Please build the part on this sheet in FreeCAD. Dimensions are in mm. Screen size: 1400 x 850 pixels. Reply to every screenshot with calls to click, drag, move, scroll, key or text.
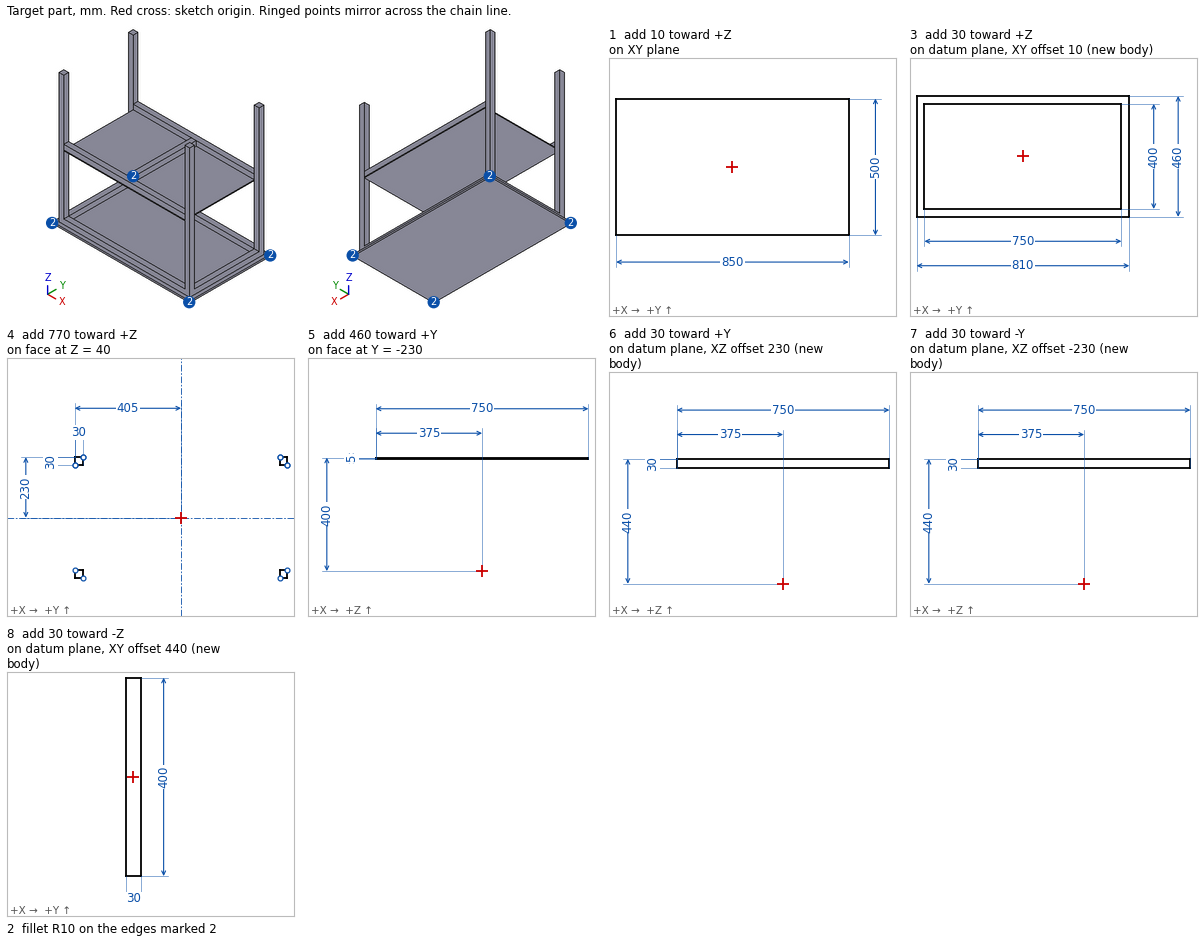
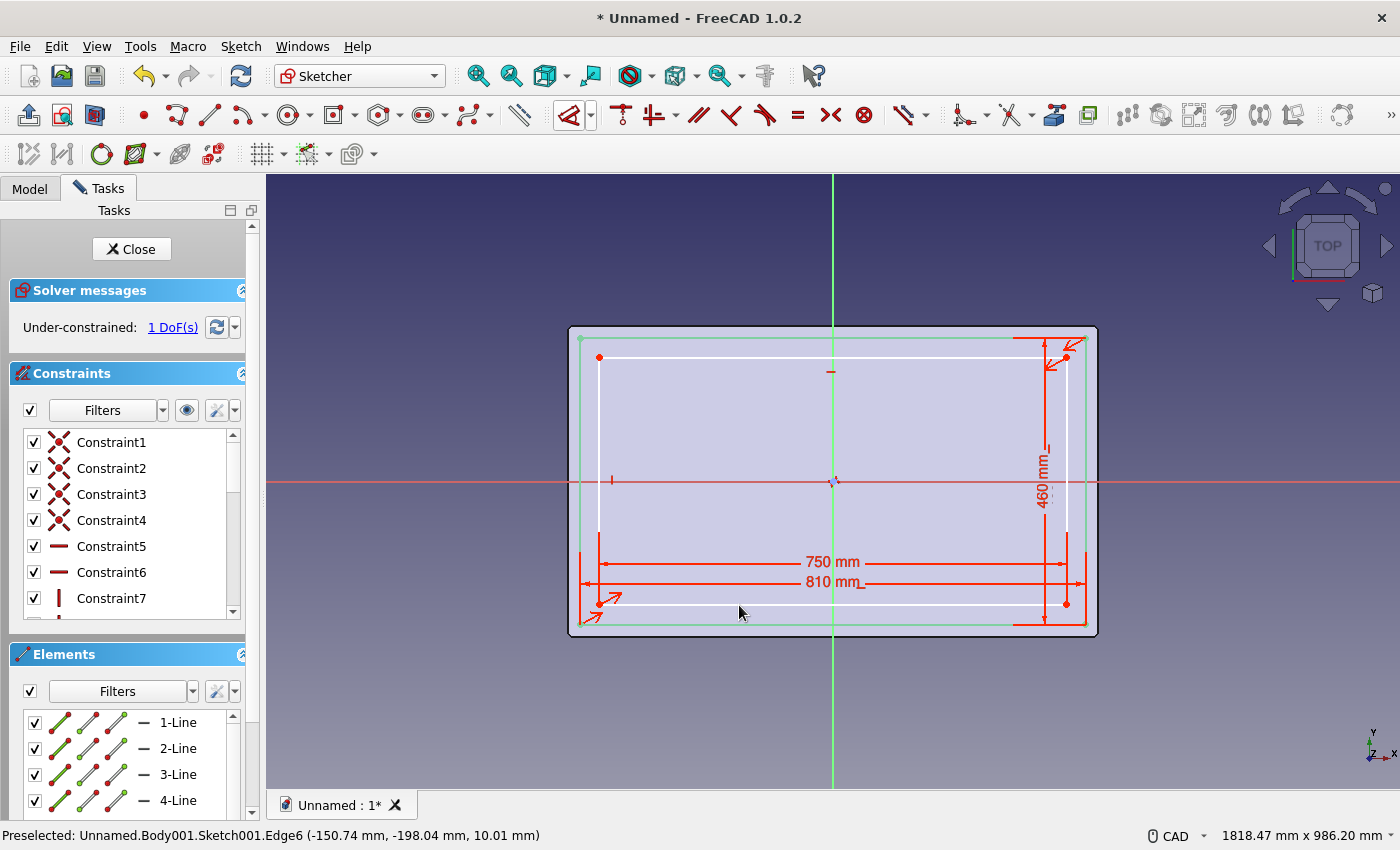
click(1067, 531)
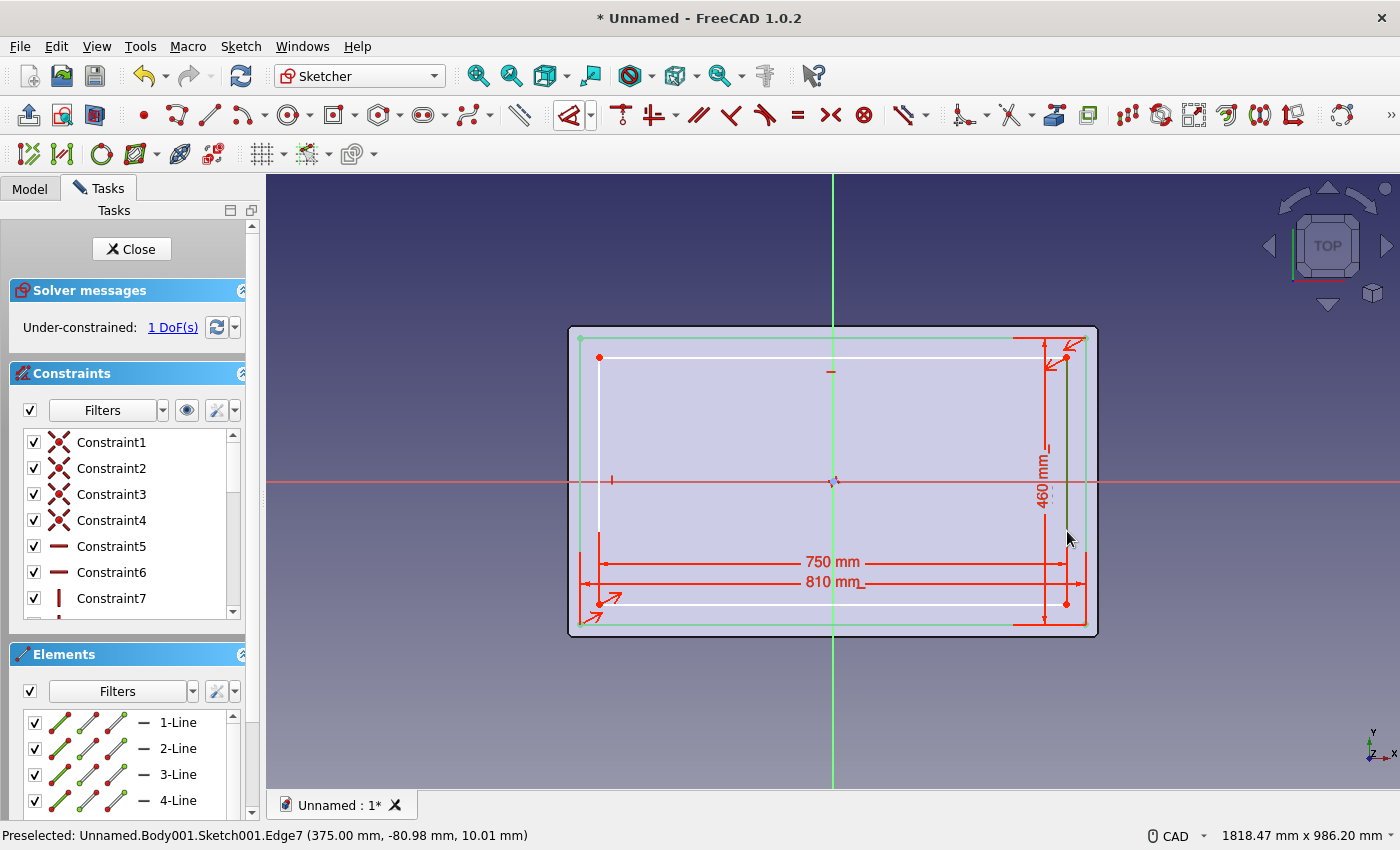
key(i)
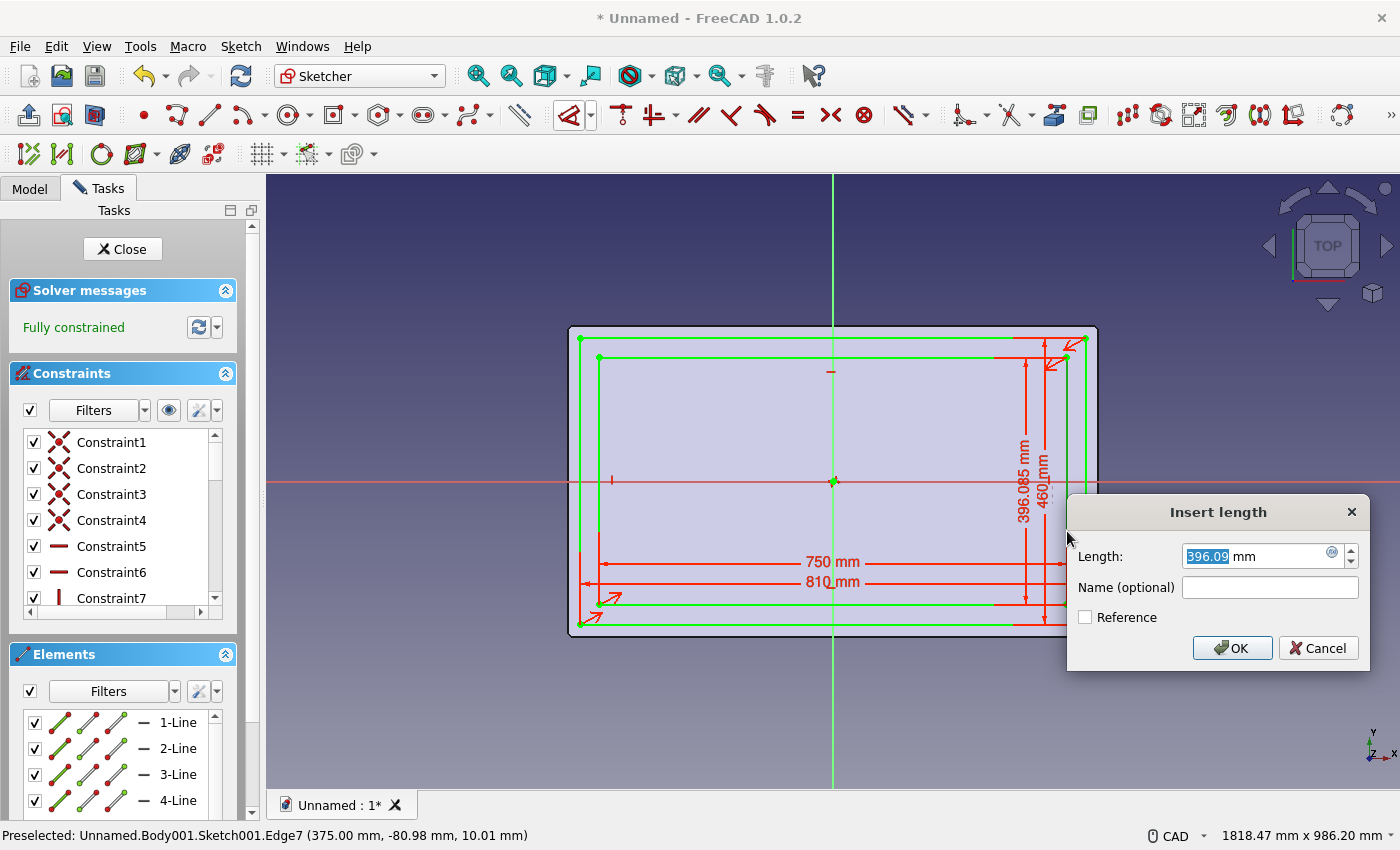
text(400)
key(Return)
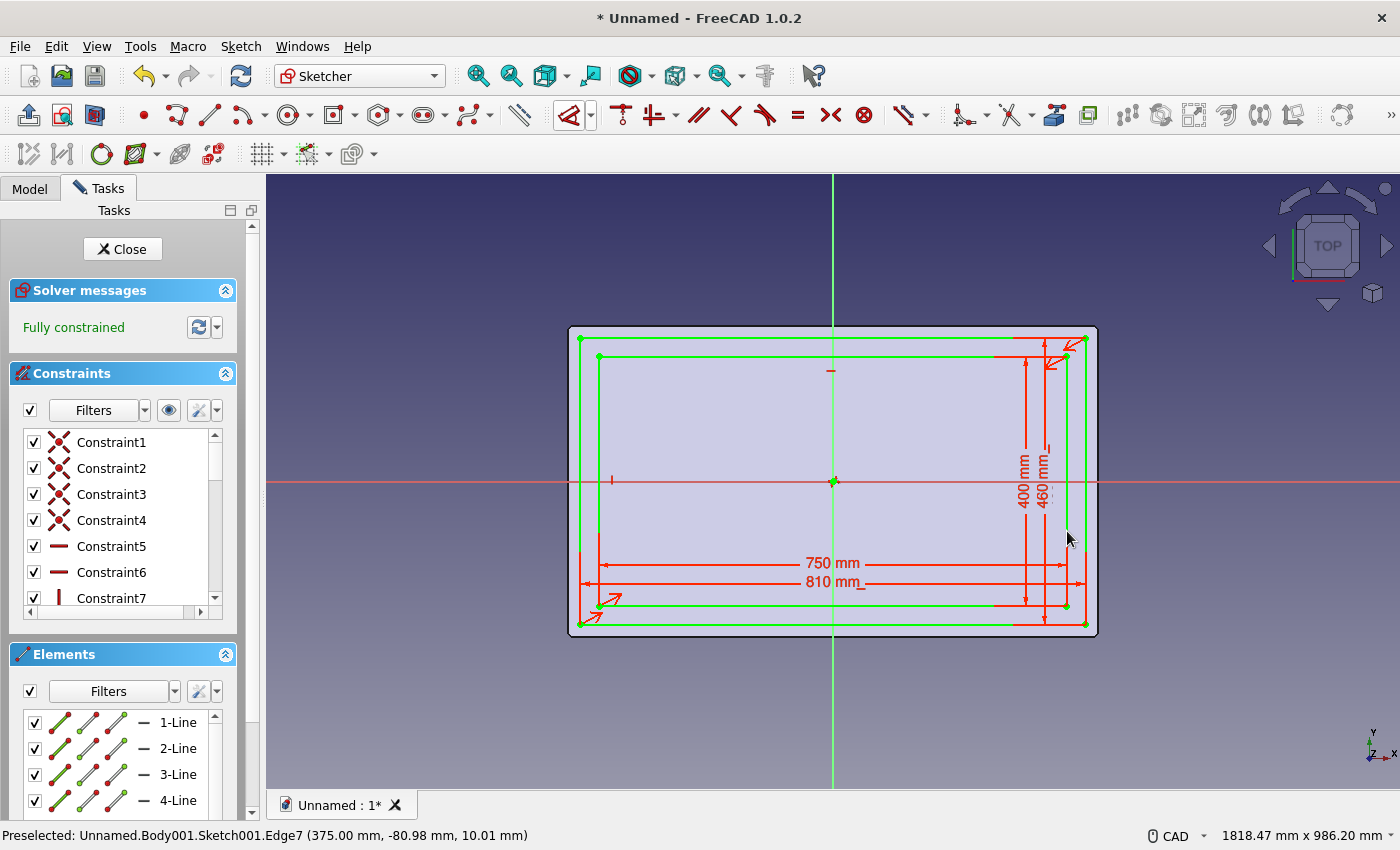
click(123, 249)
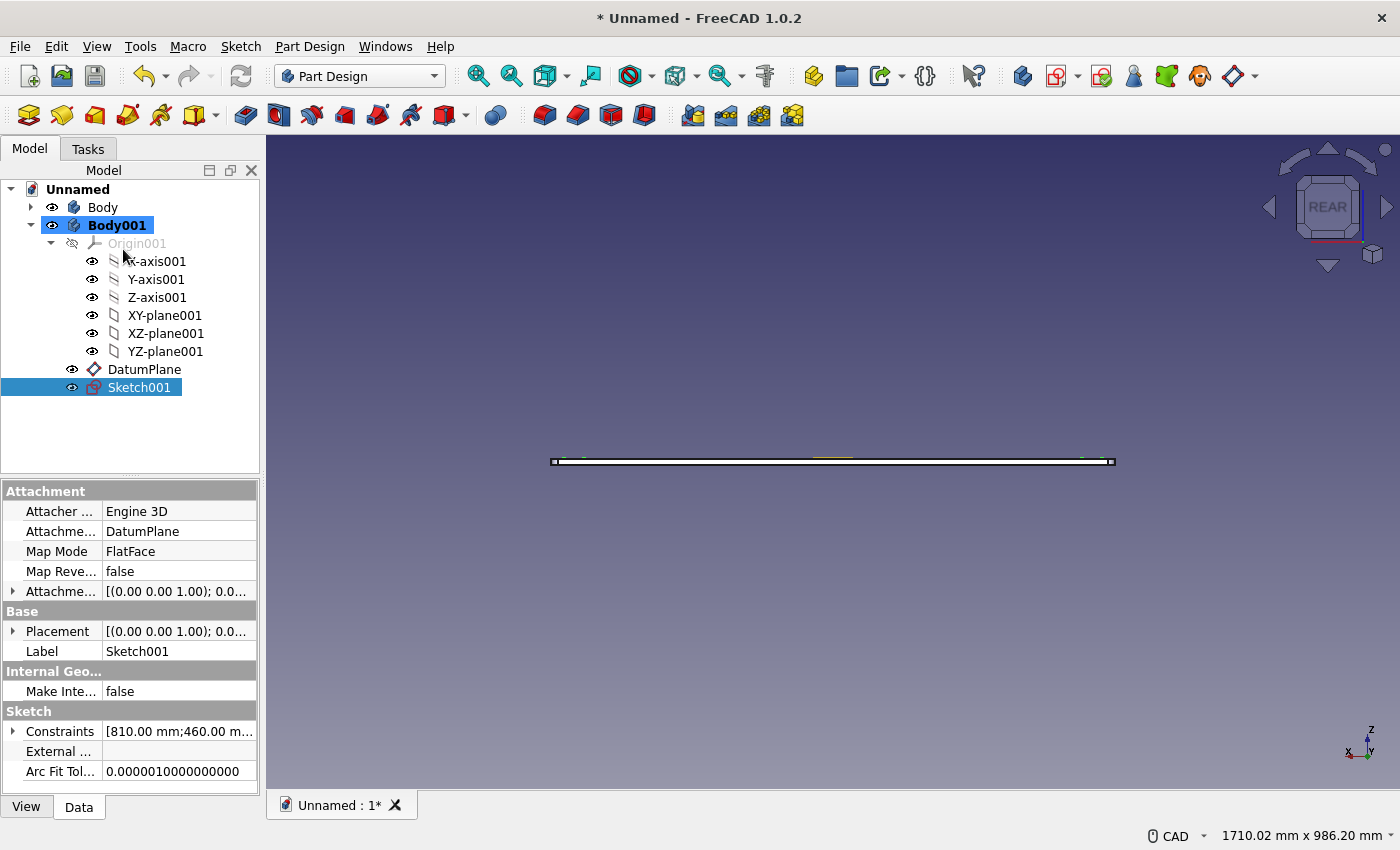
click(29, 116)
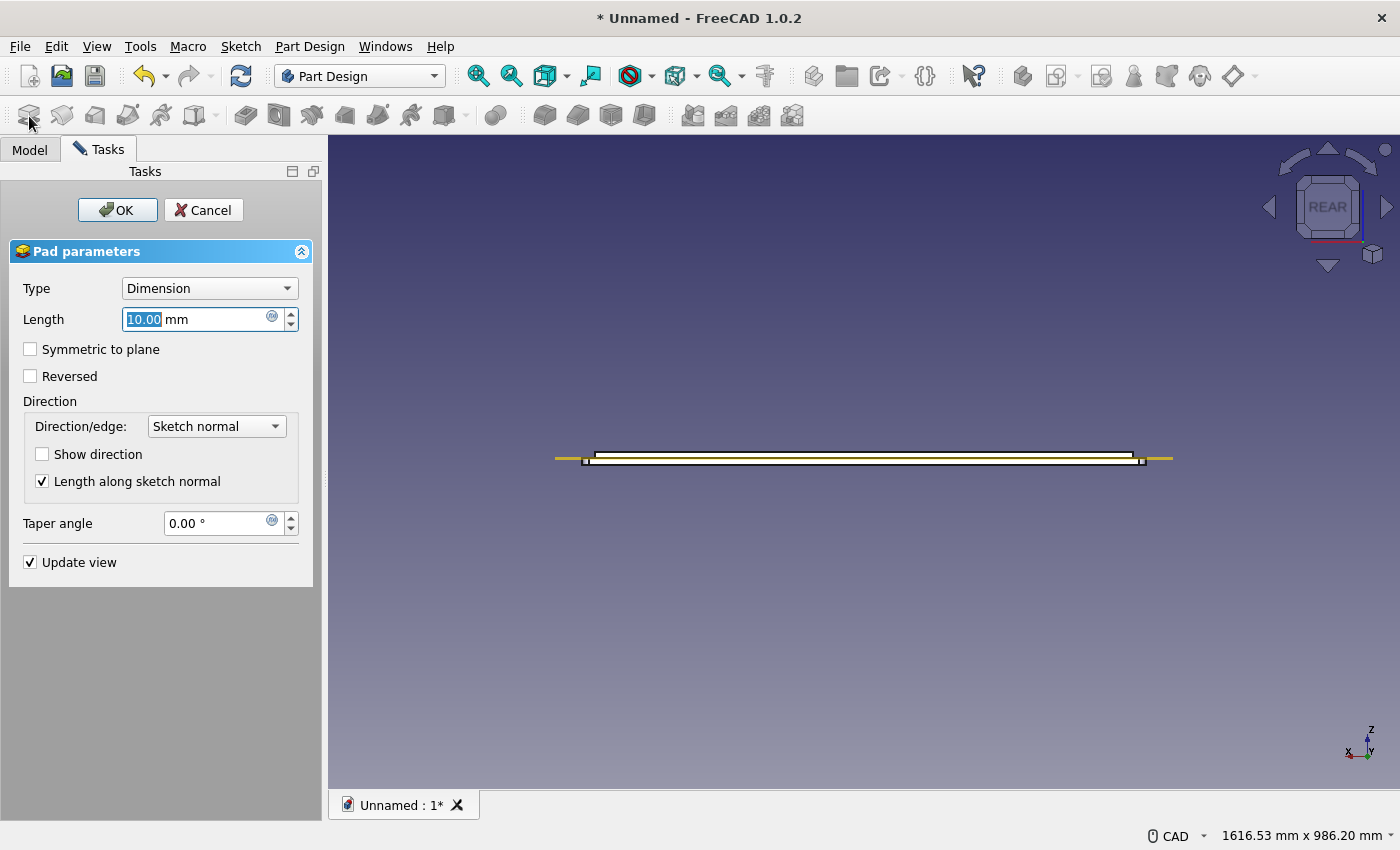
text(30)
key(Tab)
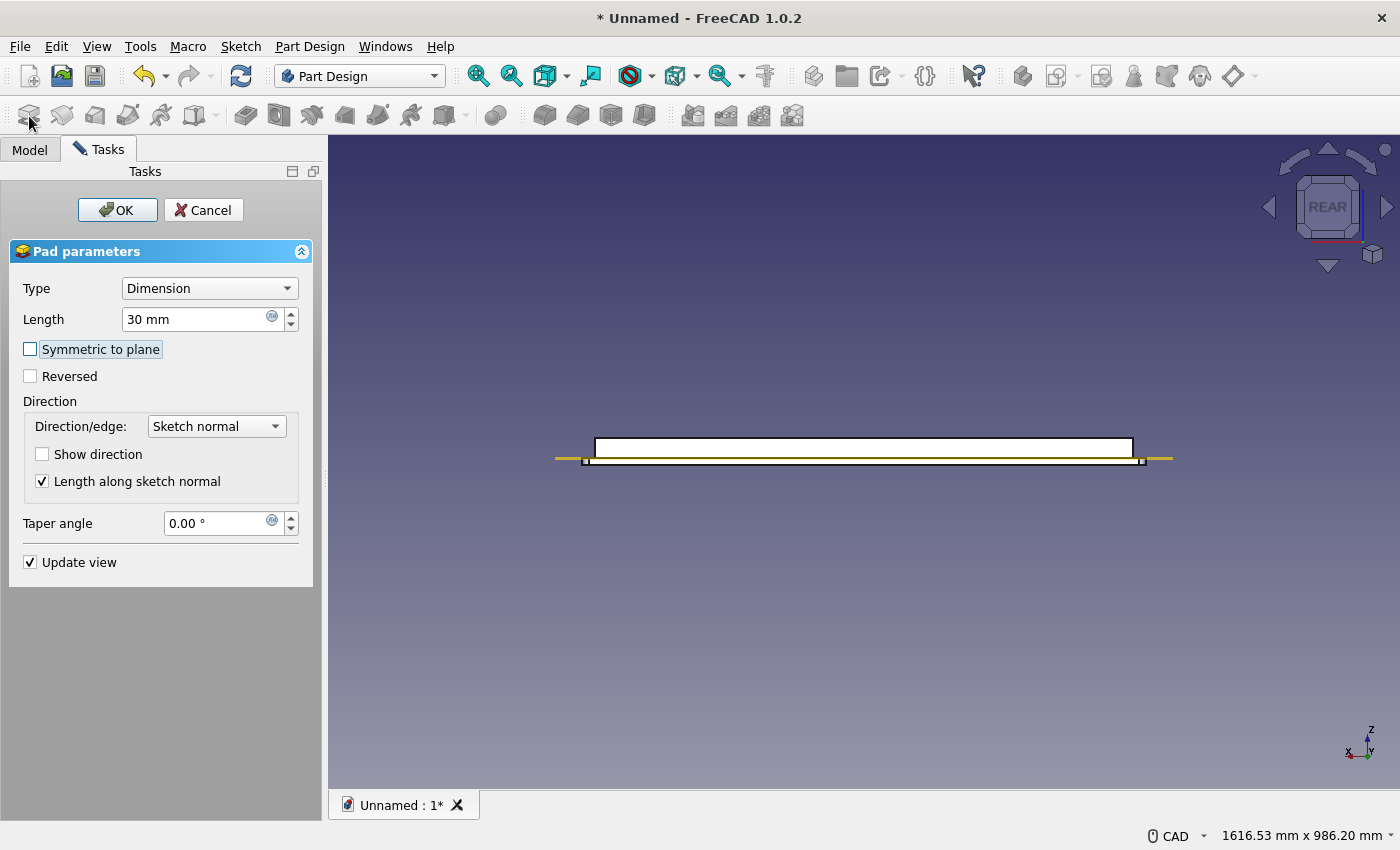
click(118, 210)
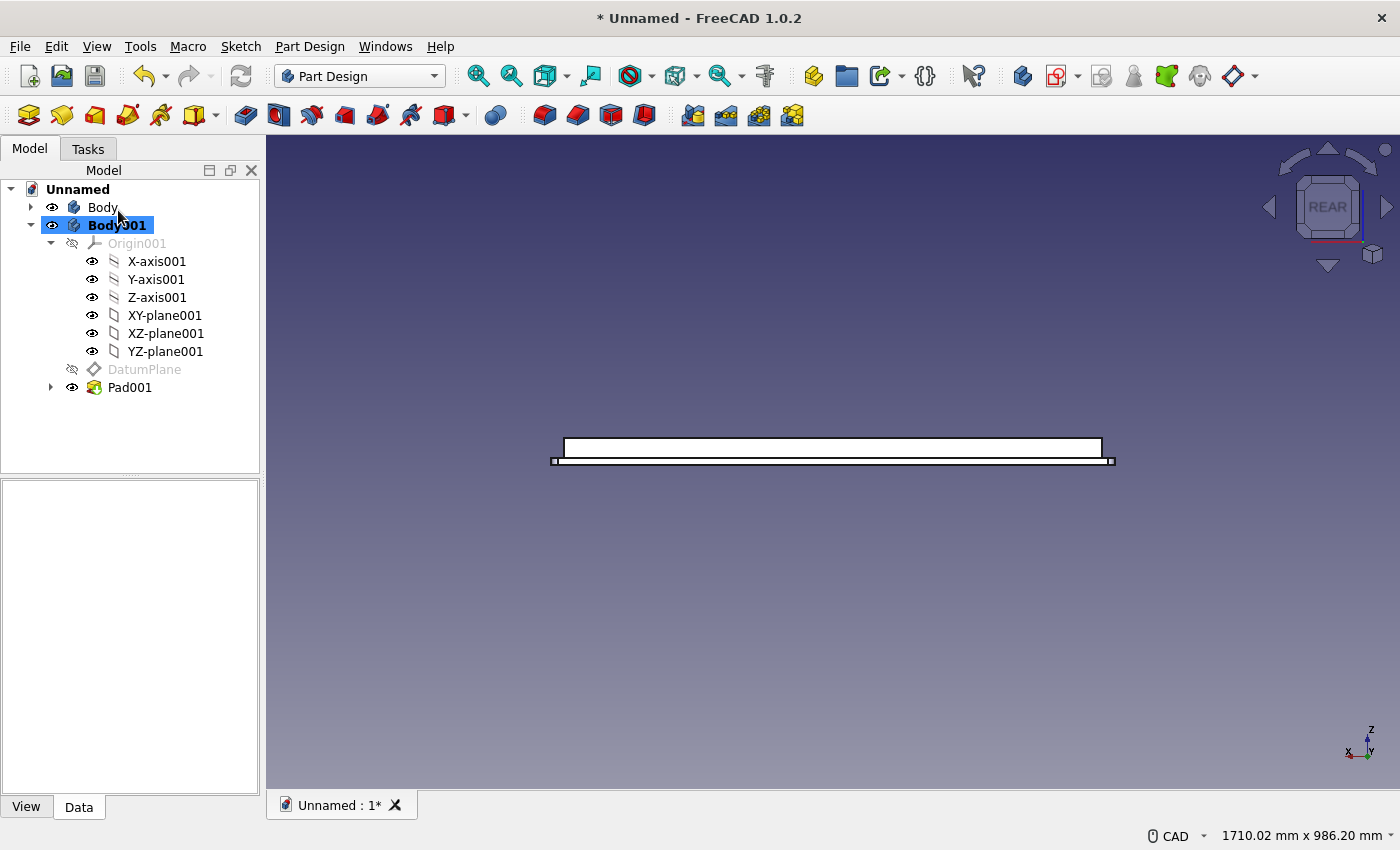
key(0)